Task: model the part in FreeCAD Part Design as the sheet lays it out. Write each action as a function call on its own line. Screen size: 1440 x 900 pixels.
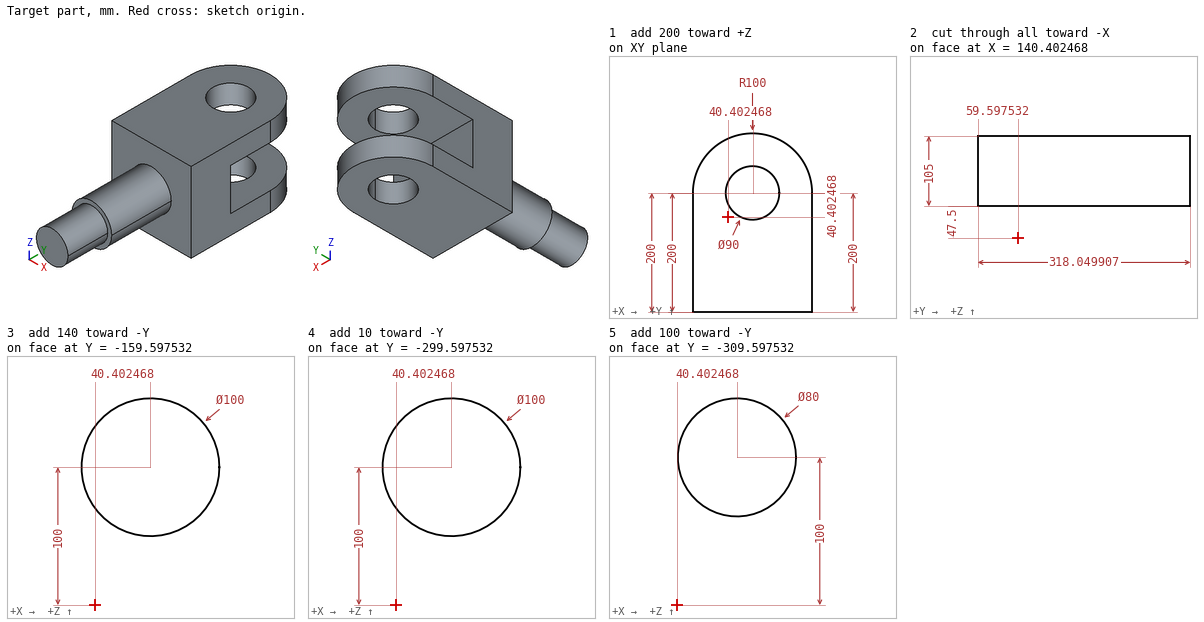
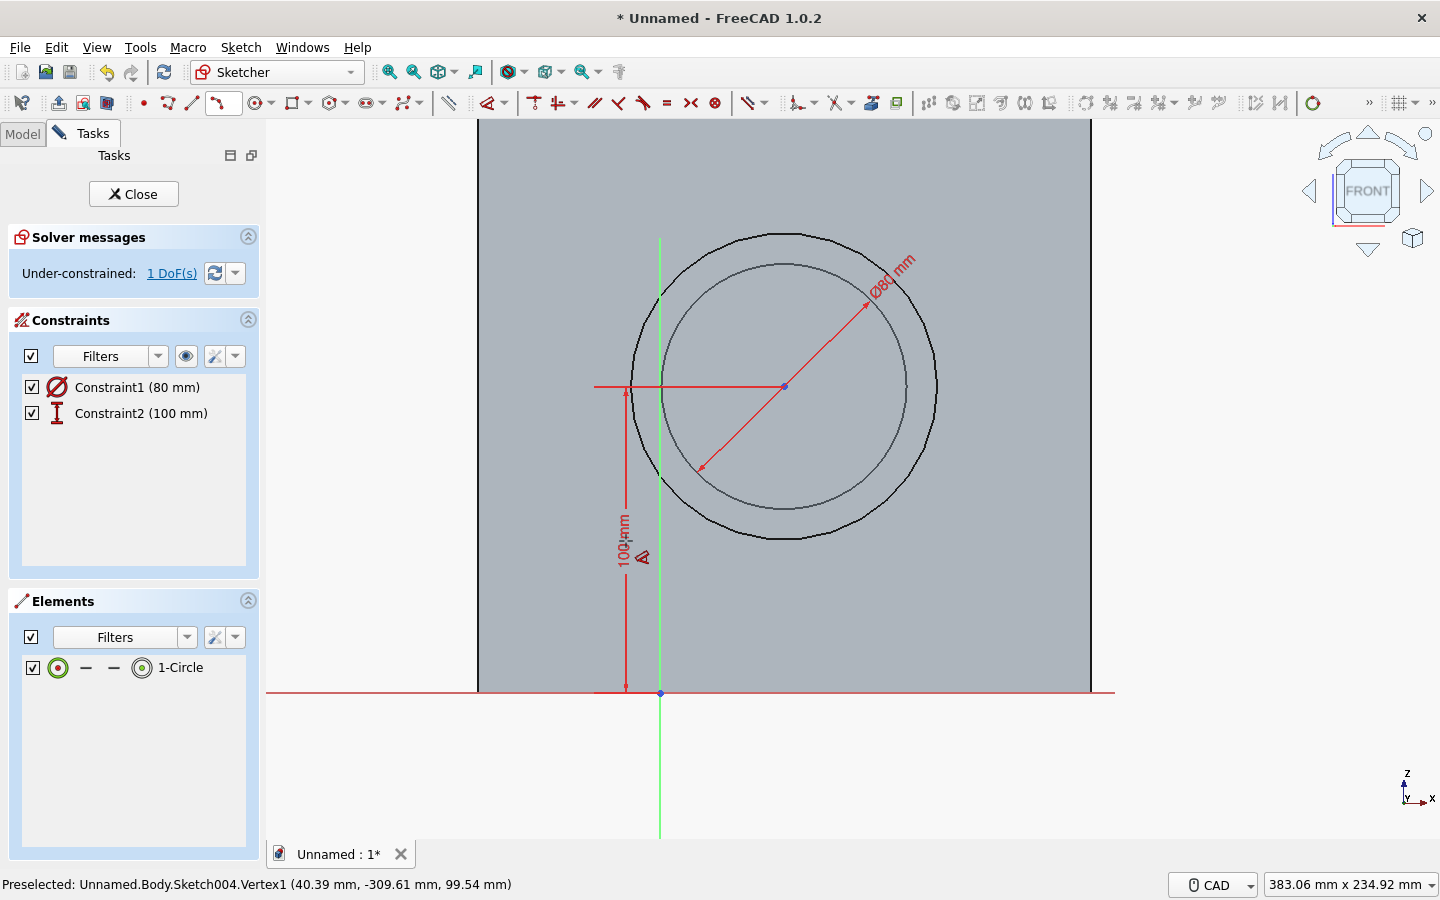
click(784, 387)
click(722, 727)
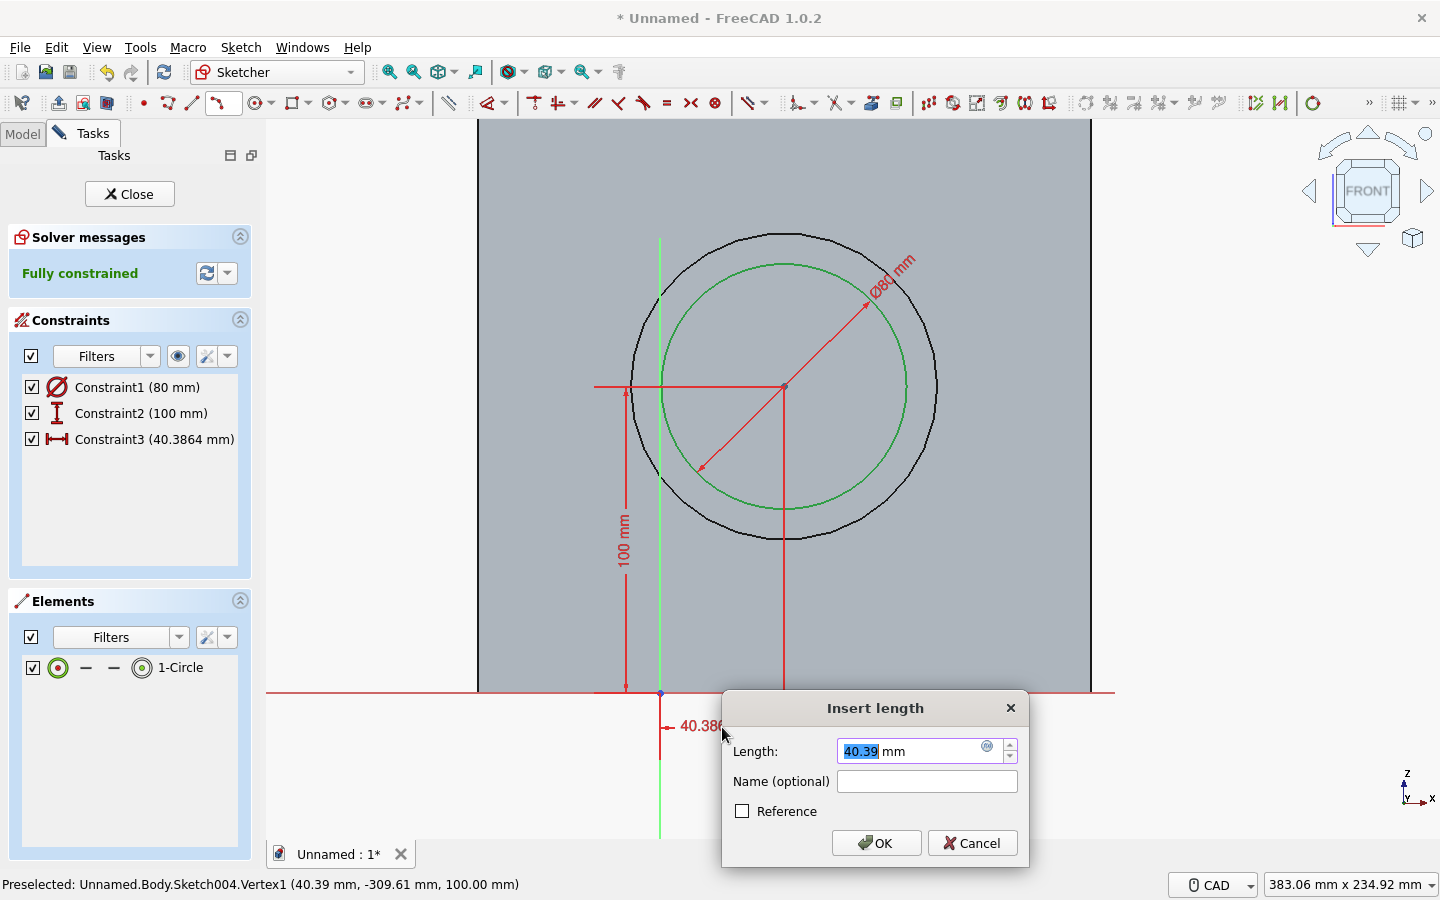
text(40.402468)
key(Return)
key(Escape)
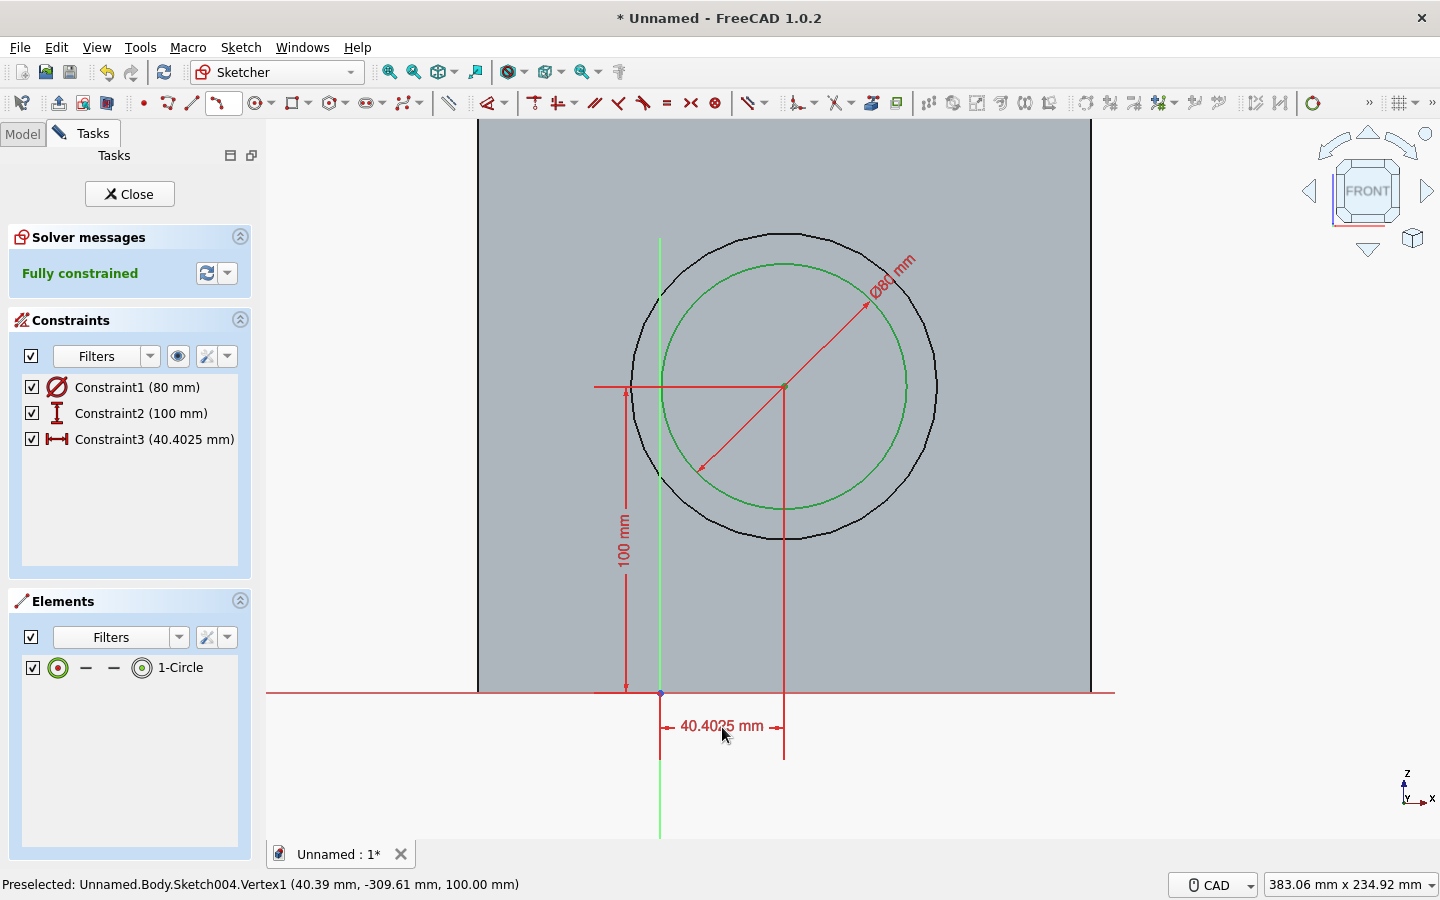
click(130, 194)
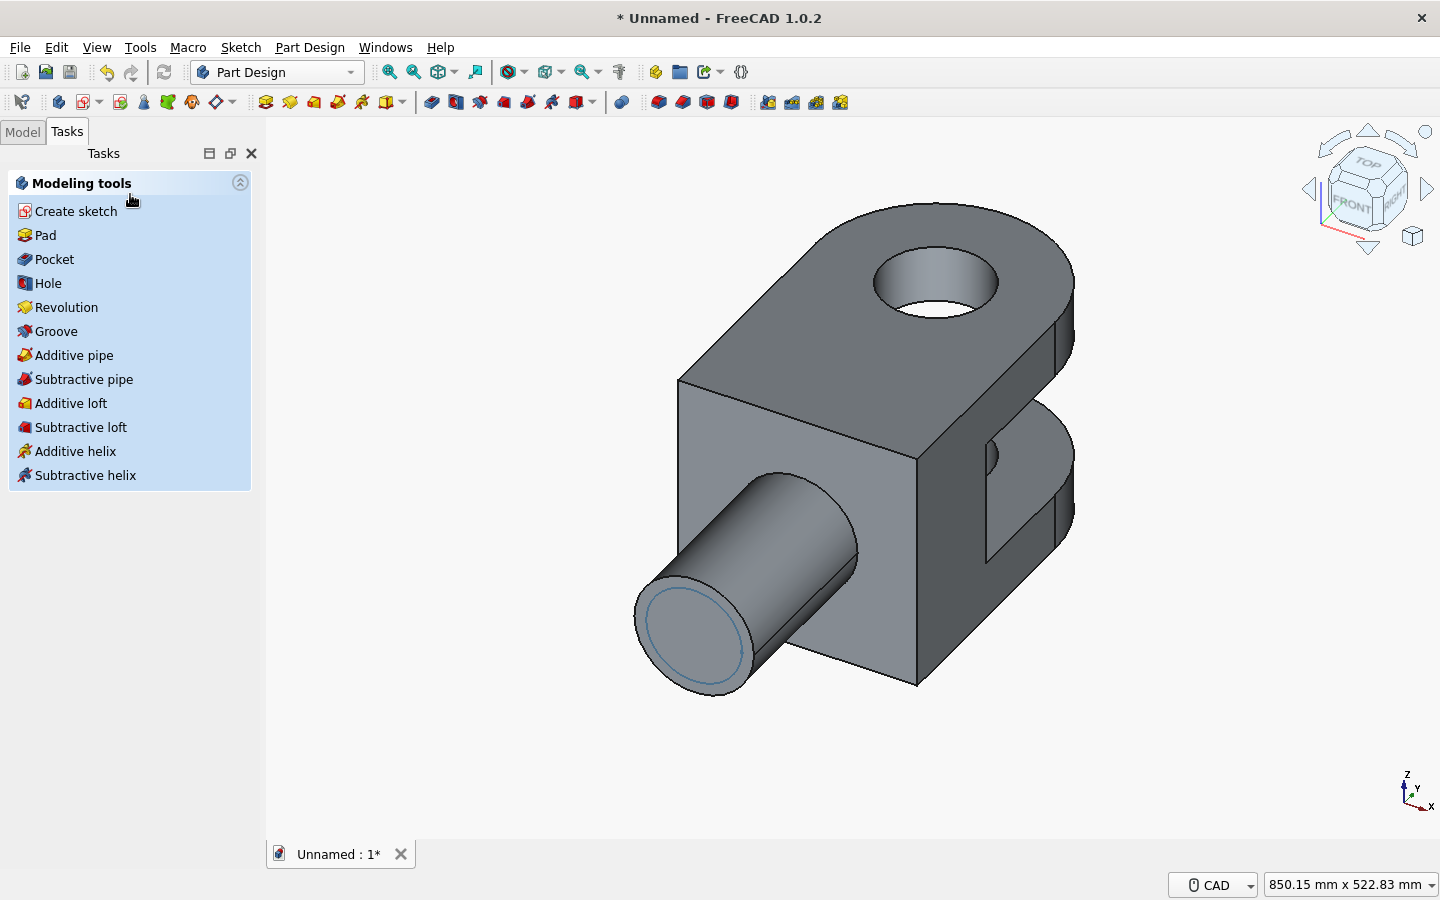
click(266, 102)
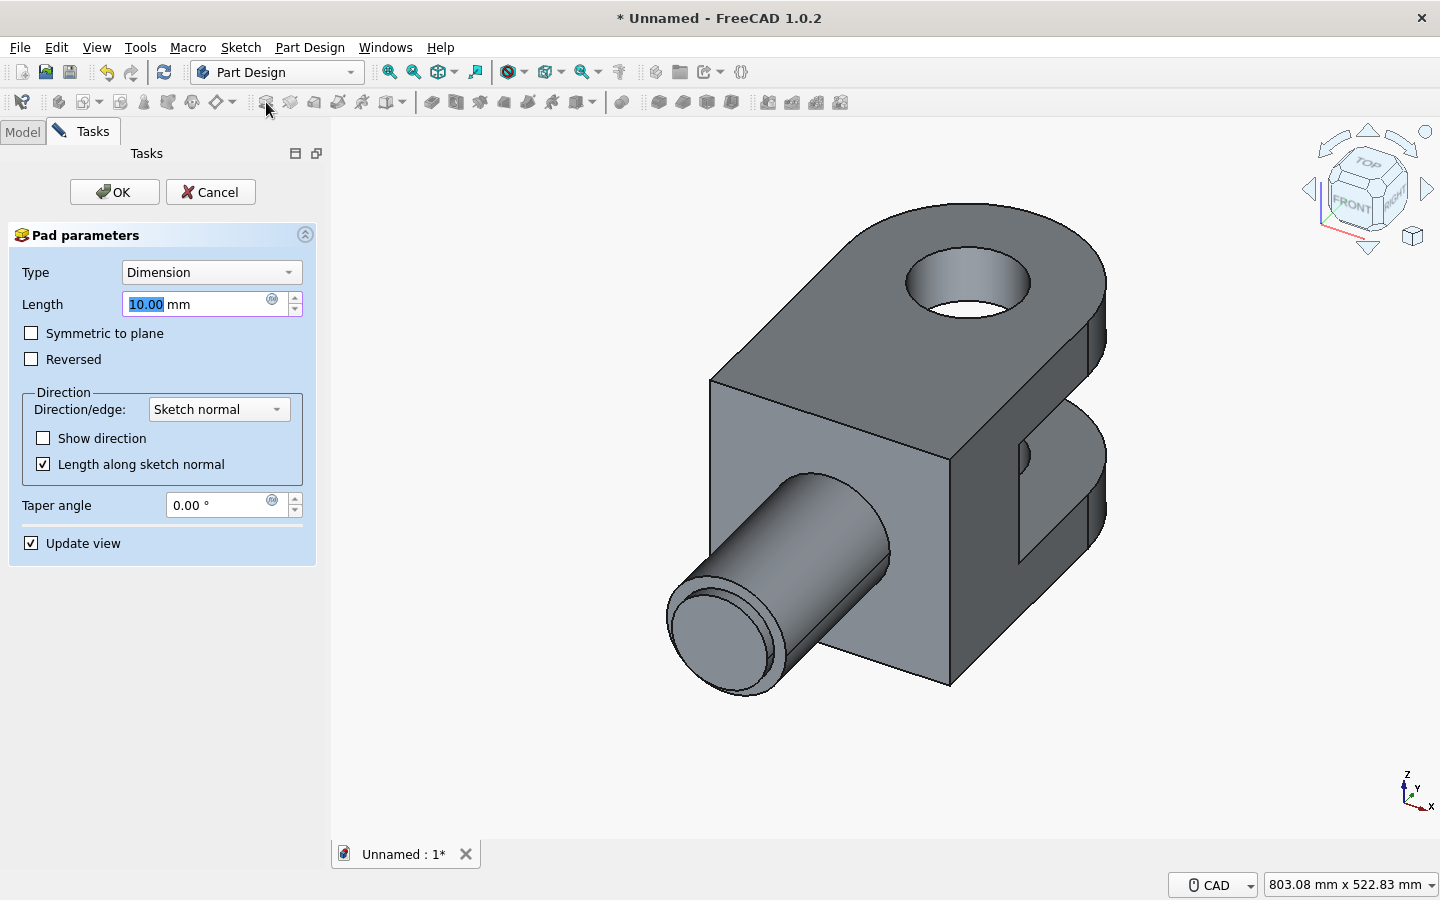
text(100)
key(Tab)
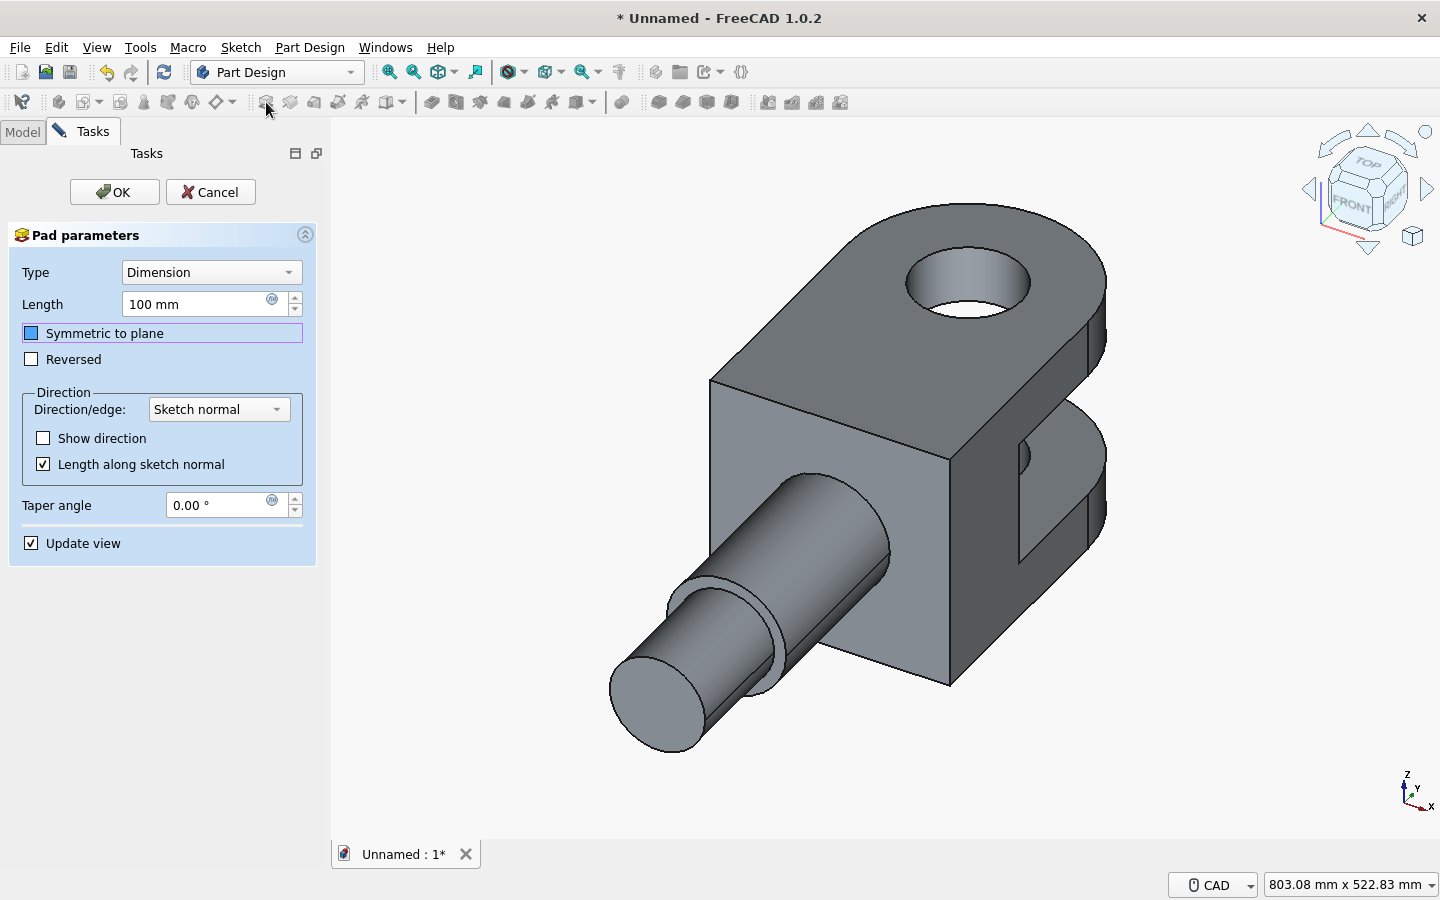
click(115, 192)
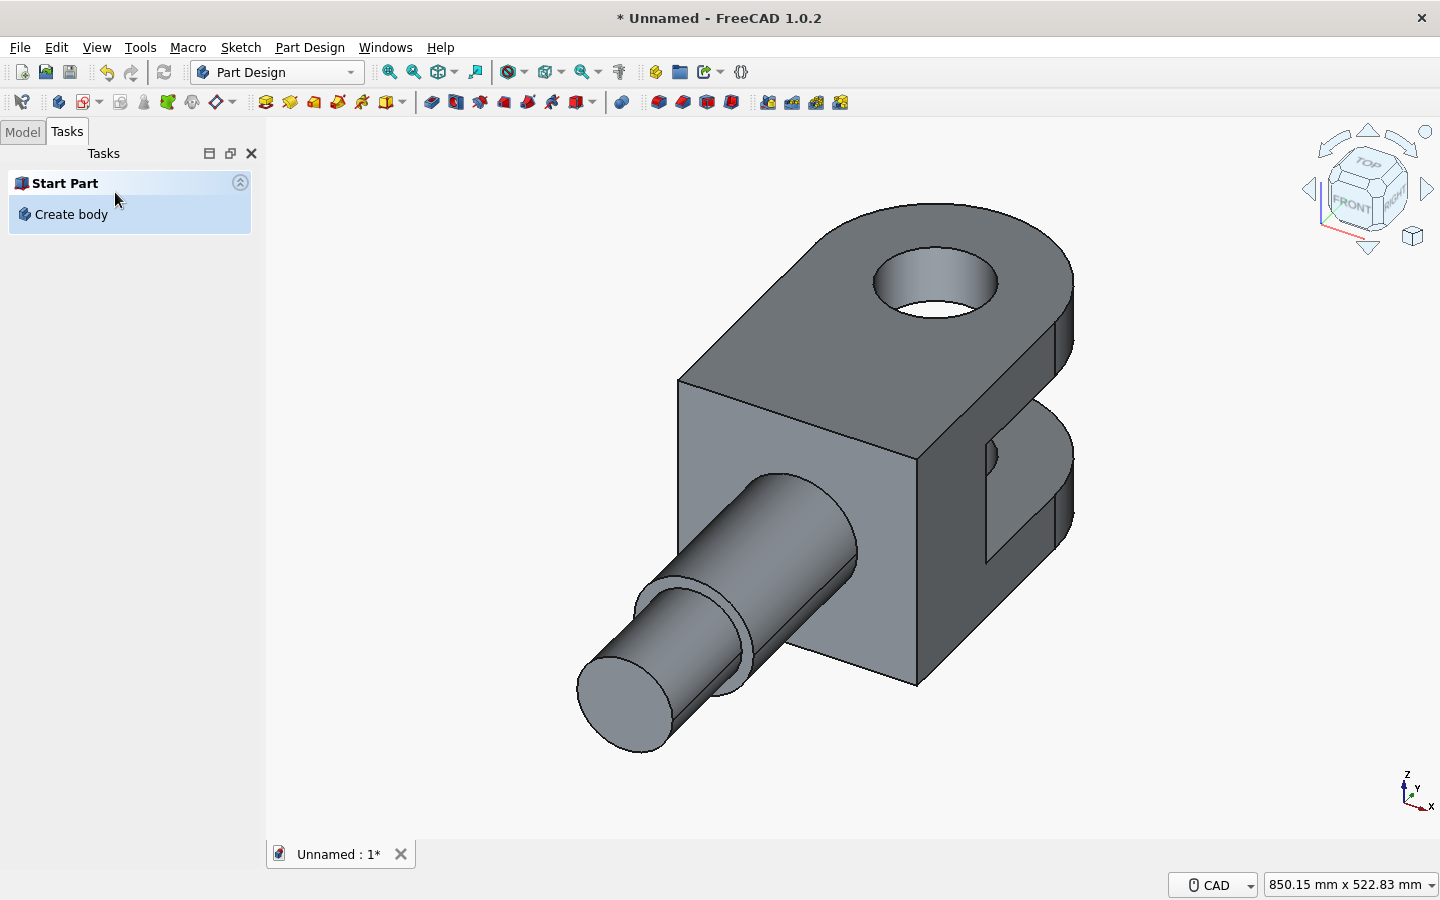
key(0)